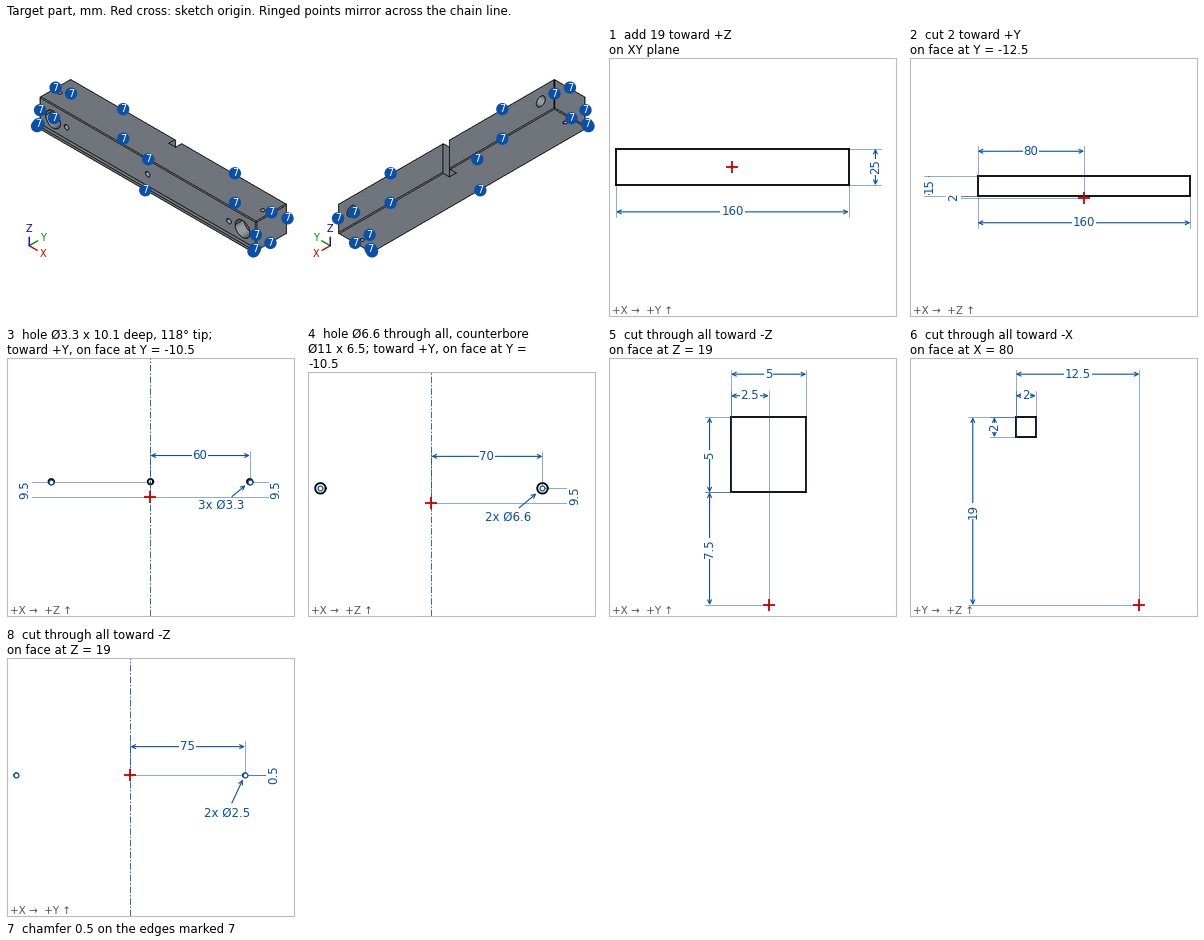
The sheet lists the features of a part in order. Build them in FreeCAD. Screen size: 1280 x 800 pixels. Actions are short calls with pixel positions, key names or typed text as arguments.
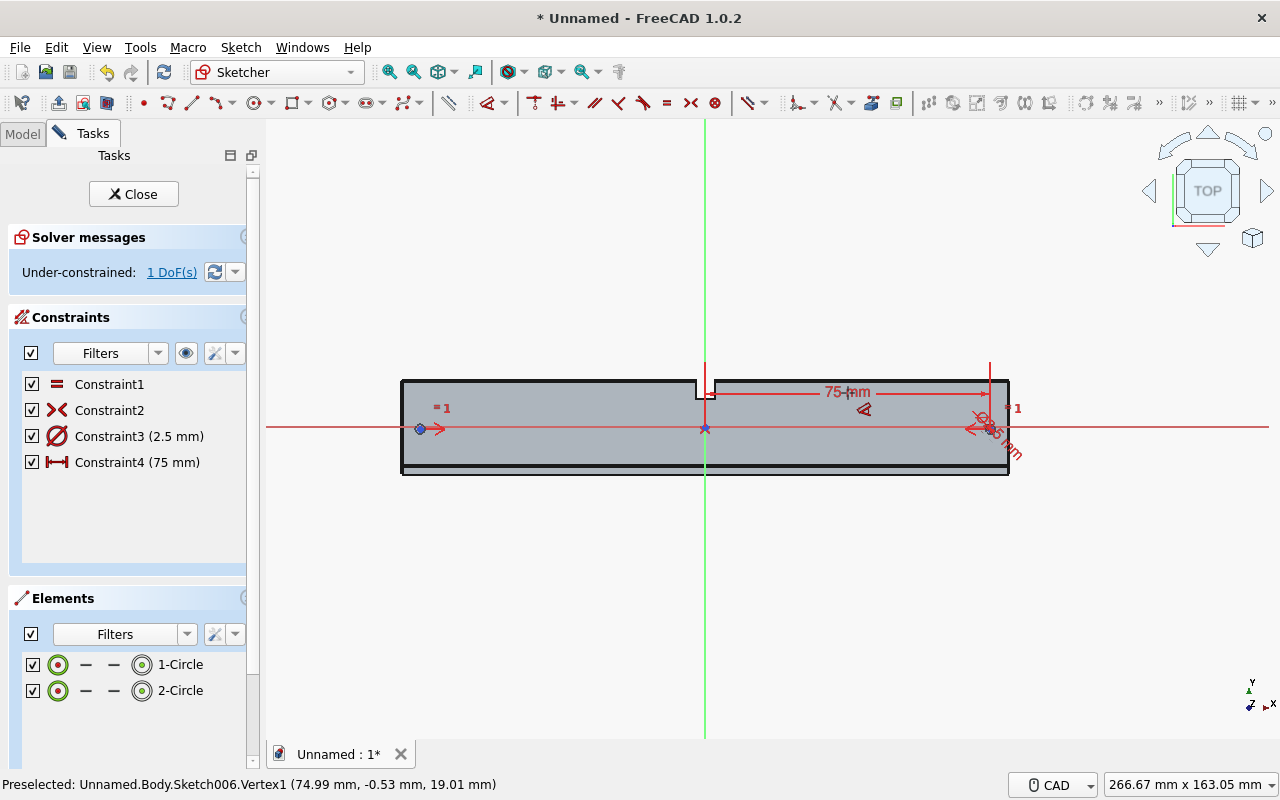
scroll(990, 429, up, 16)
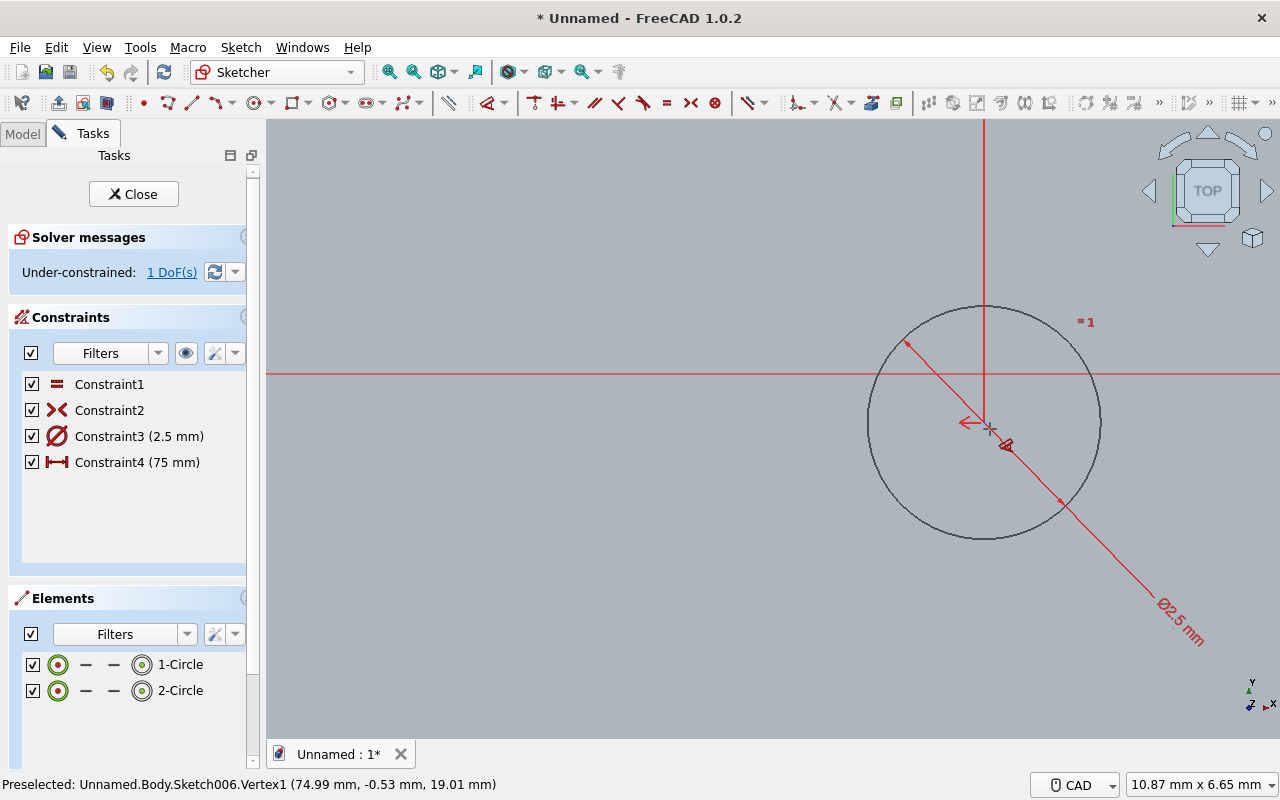
click(984, 423)
click(1018, 398)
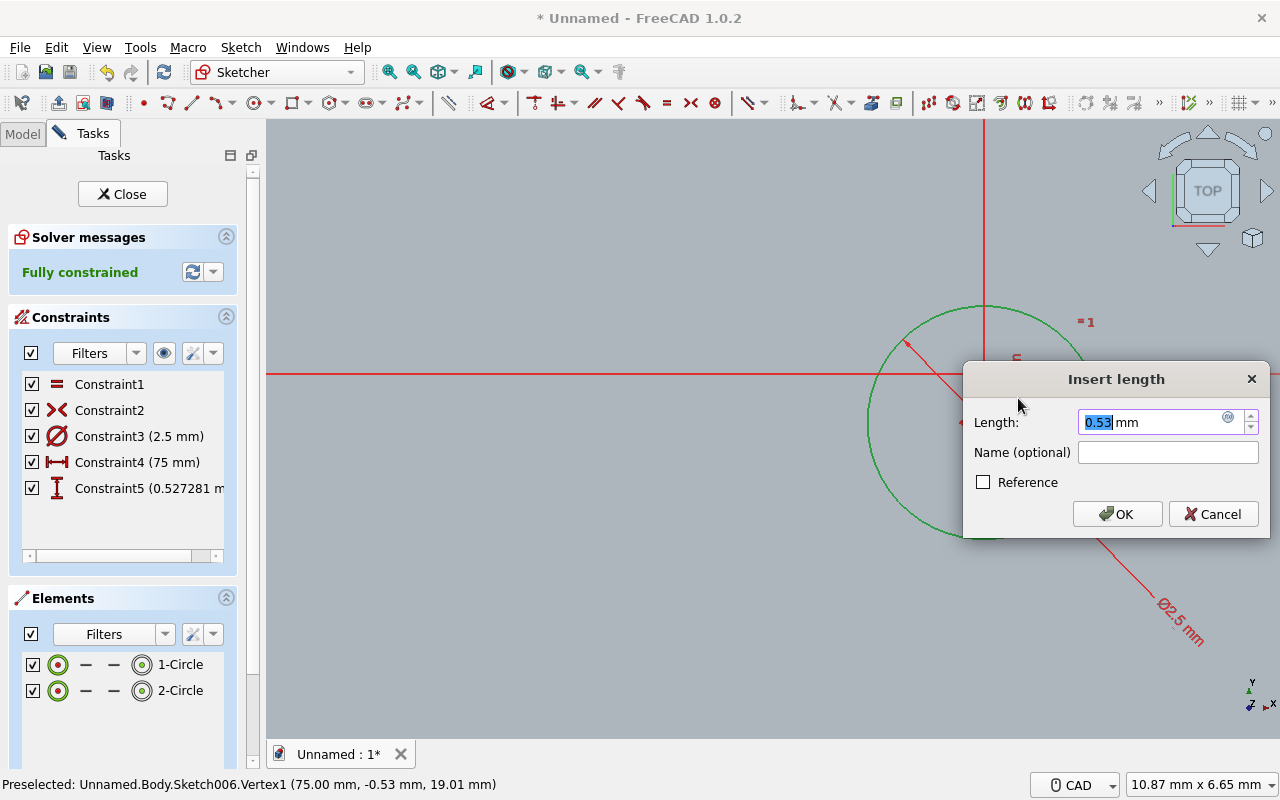
text(0.5)
key(Return)
key(Escape)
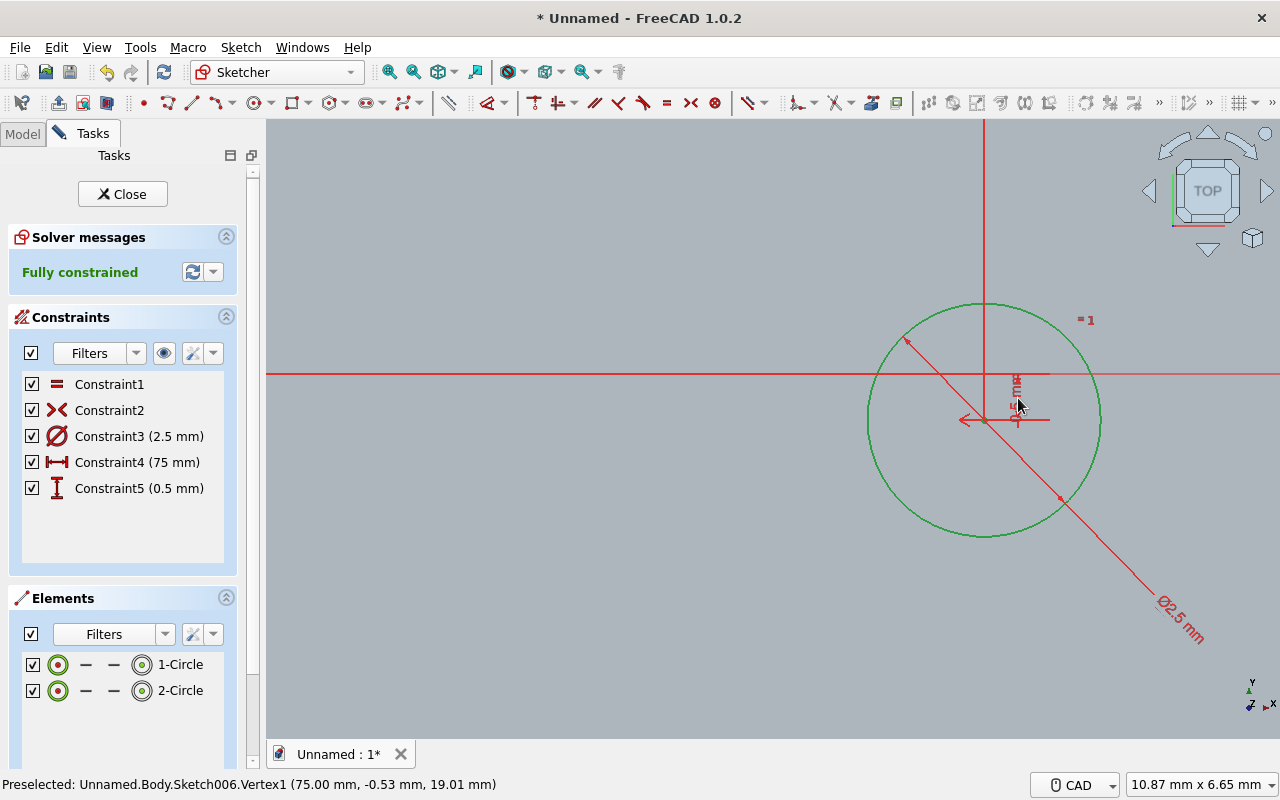
click(123, 194)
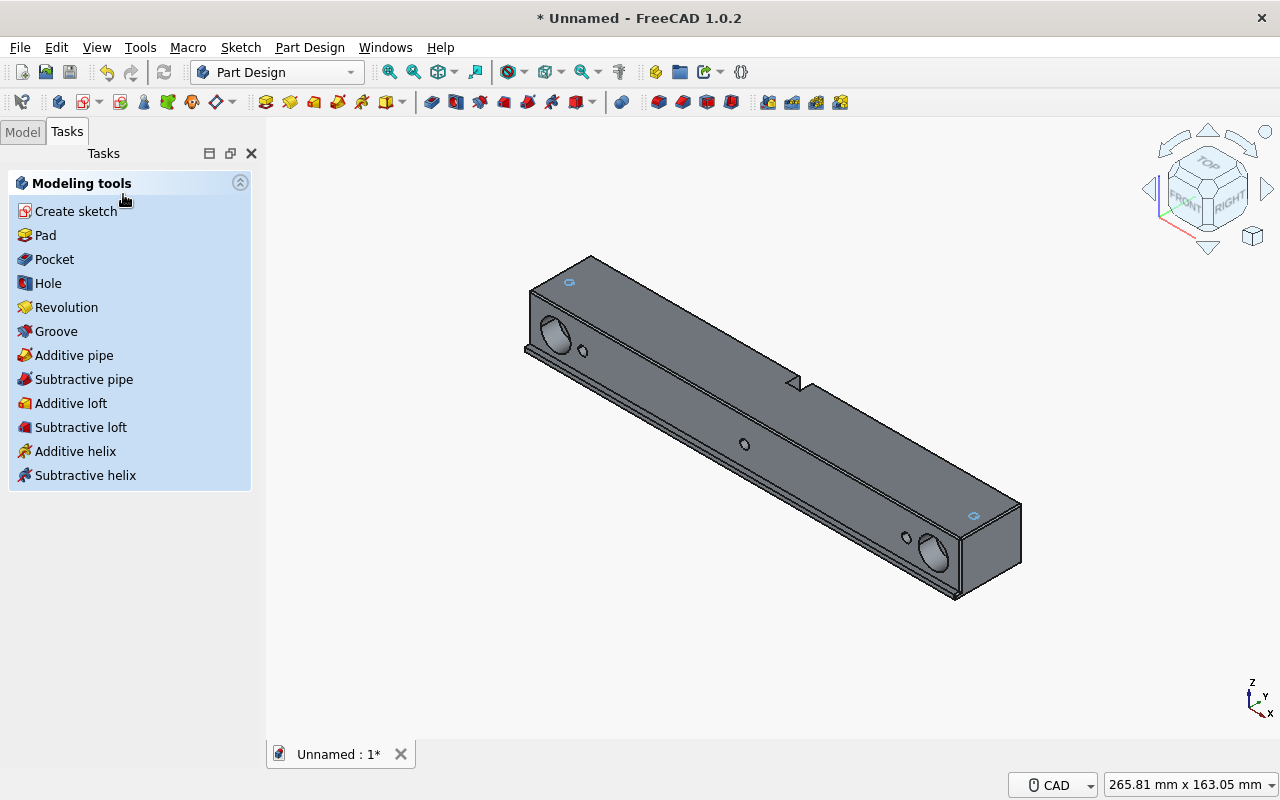
click(432, 102)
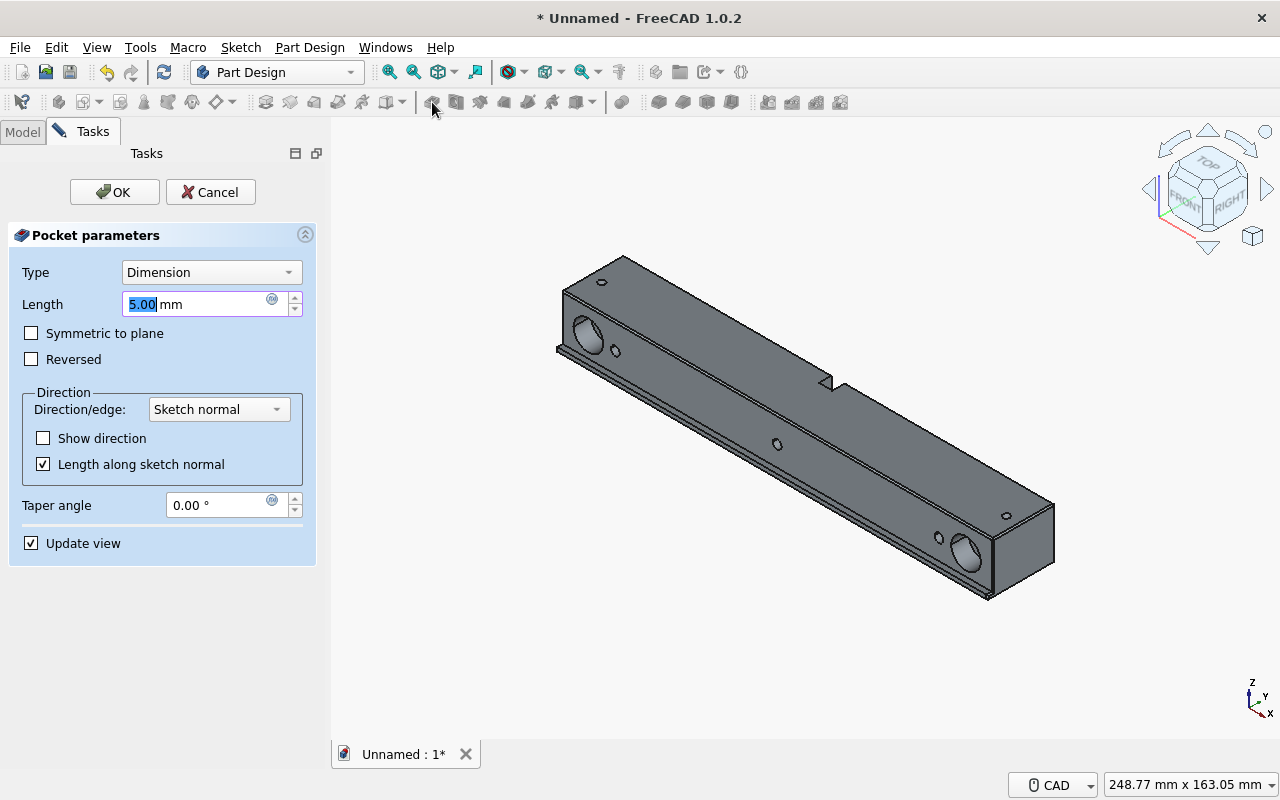
click(212, 272)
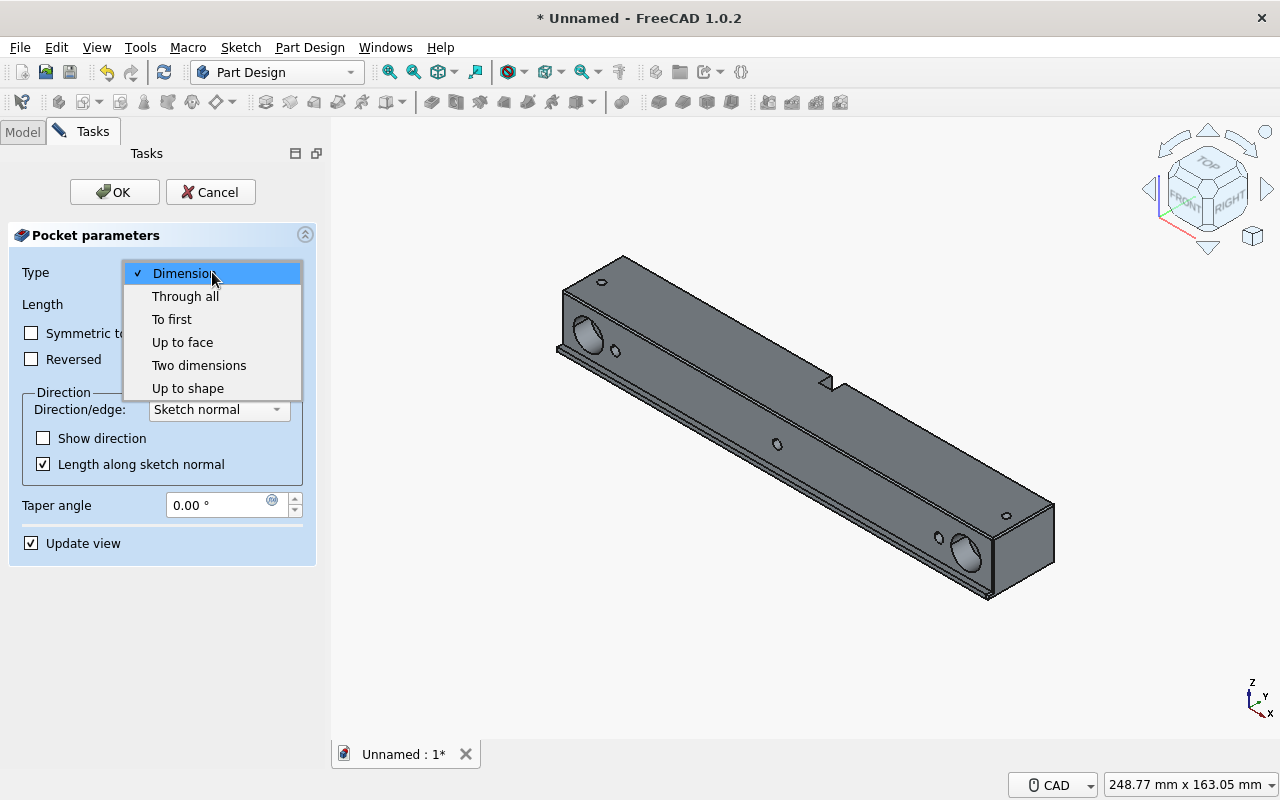
click(212, 296)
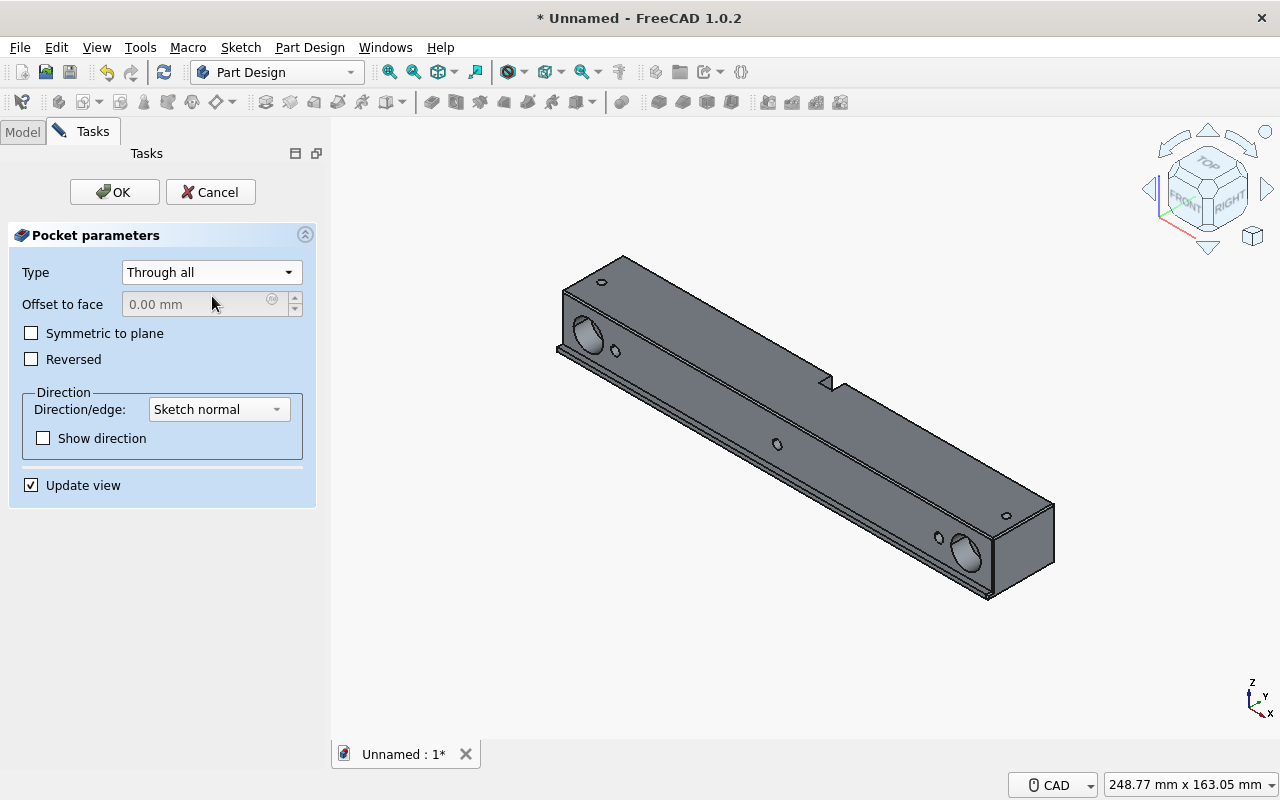
click(115, 192)